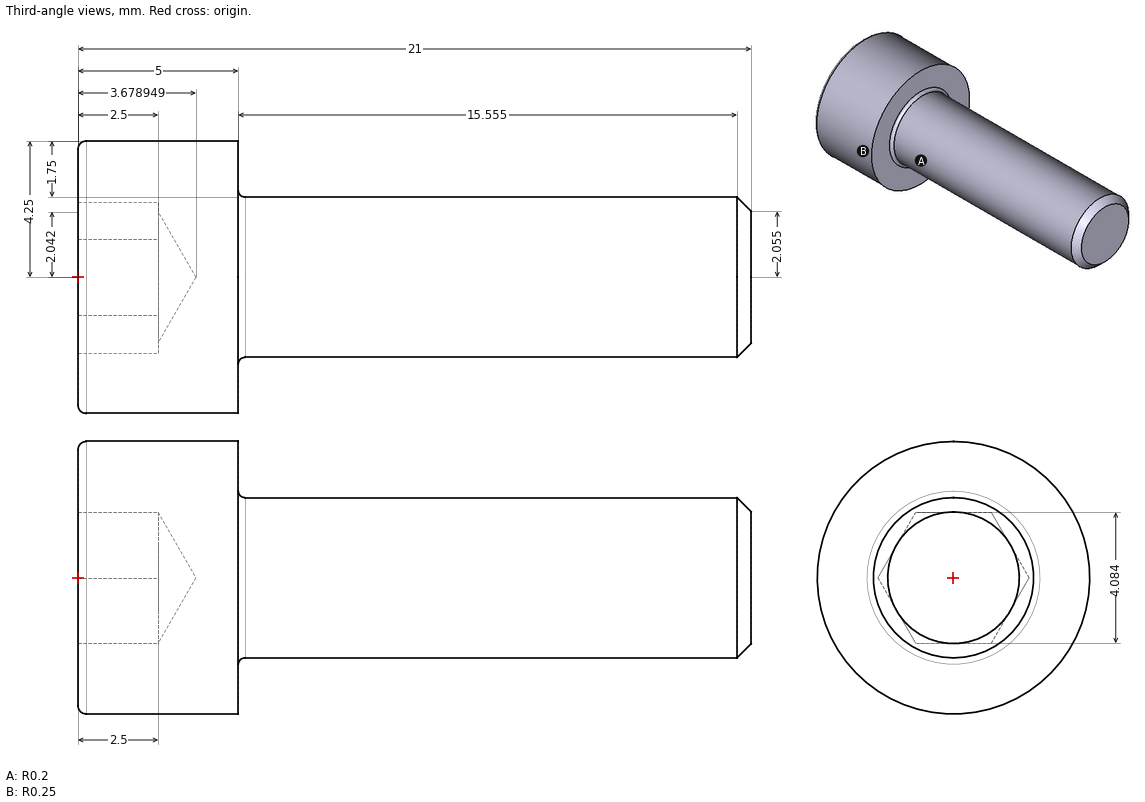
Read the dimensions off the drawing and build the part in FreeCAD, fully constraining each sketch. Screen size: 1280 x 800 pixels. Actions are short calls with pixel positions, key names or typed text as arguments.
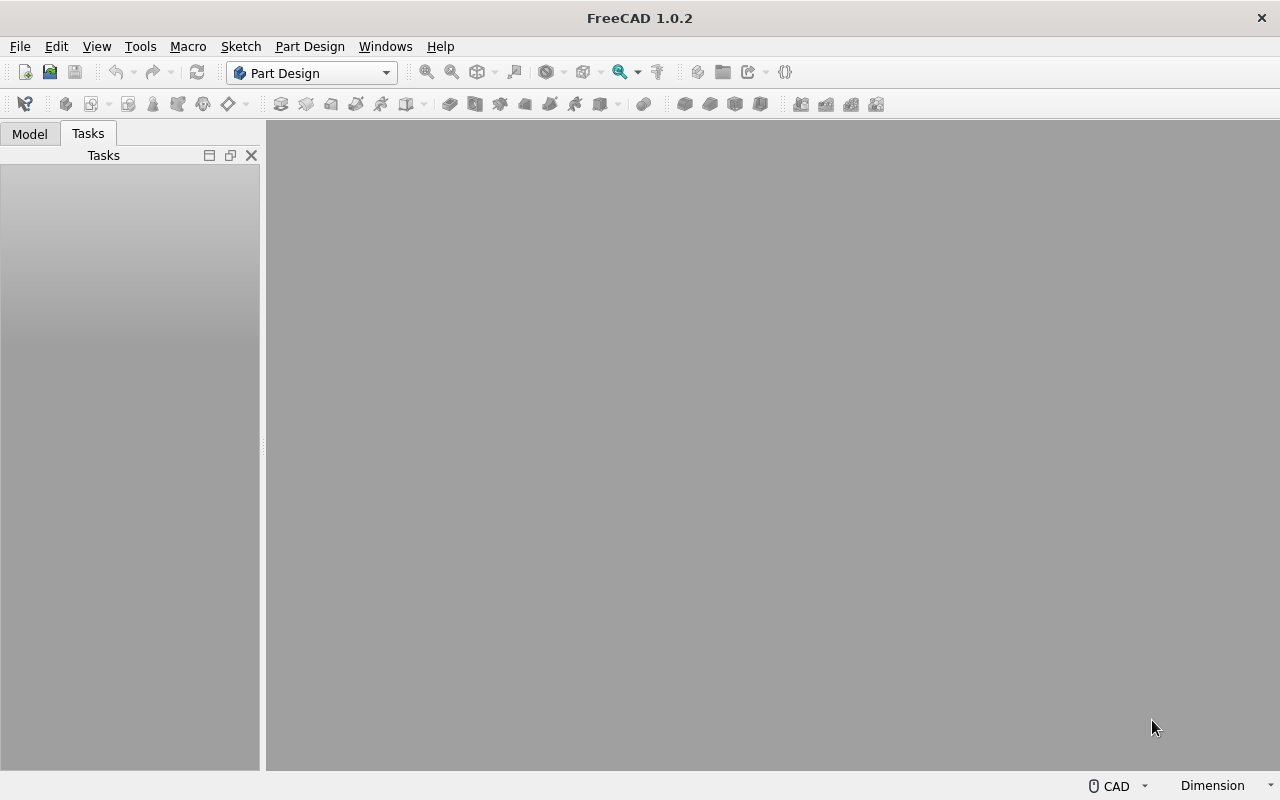
click(25, 72)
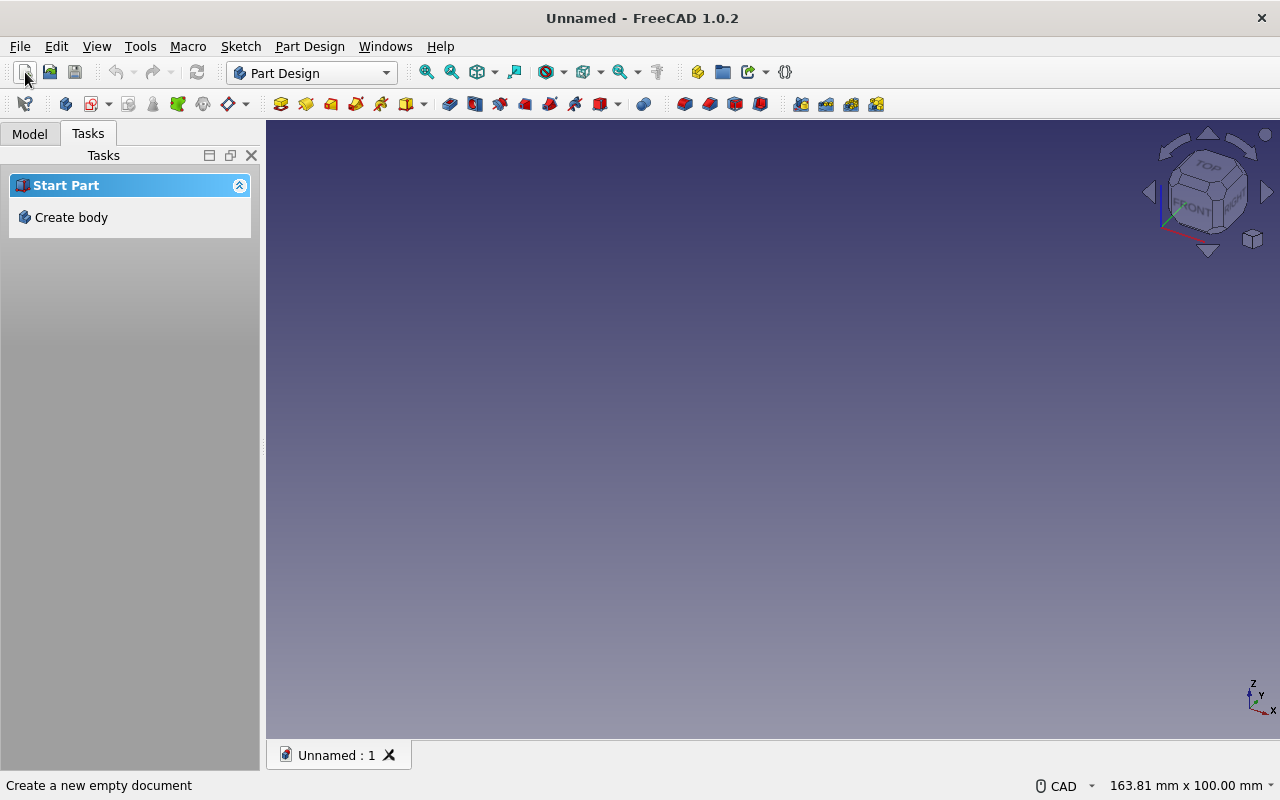
click(90, 104)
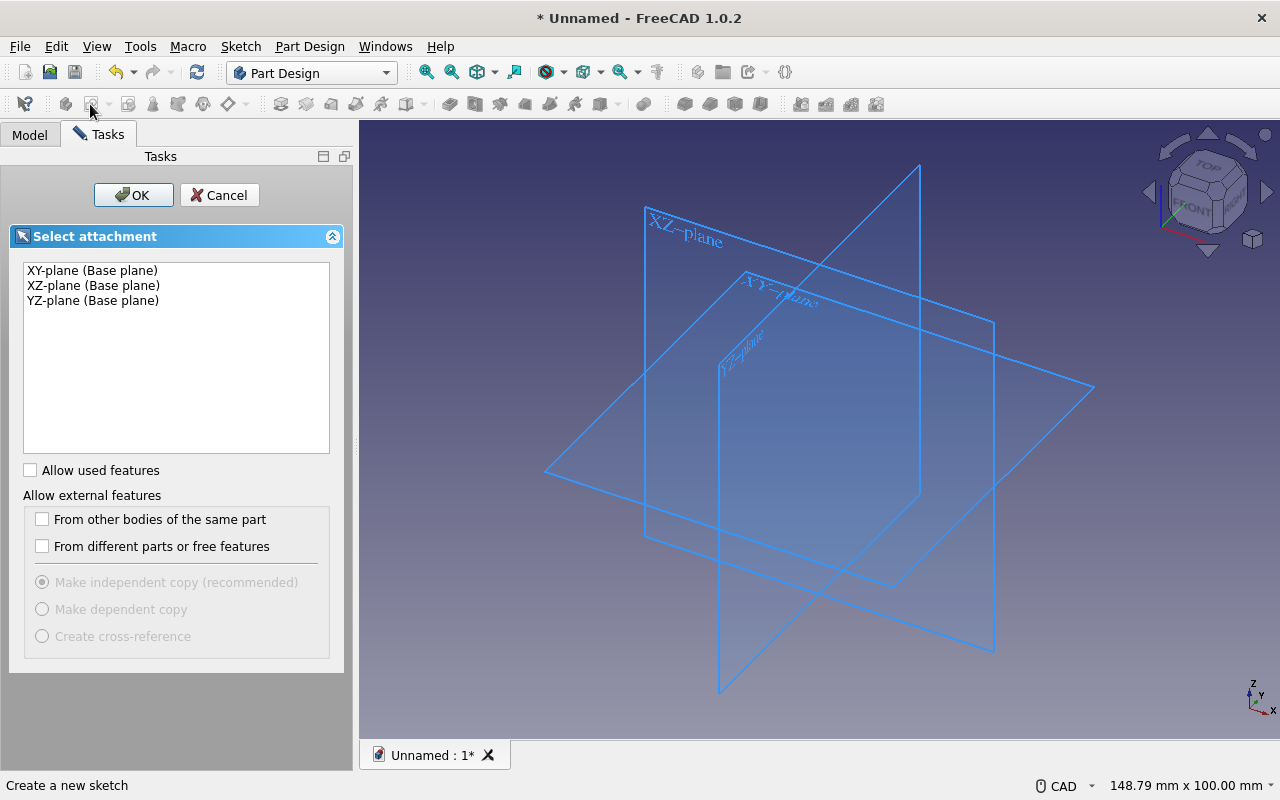
click(84, 270)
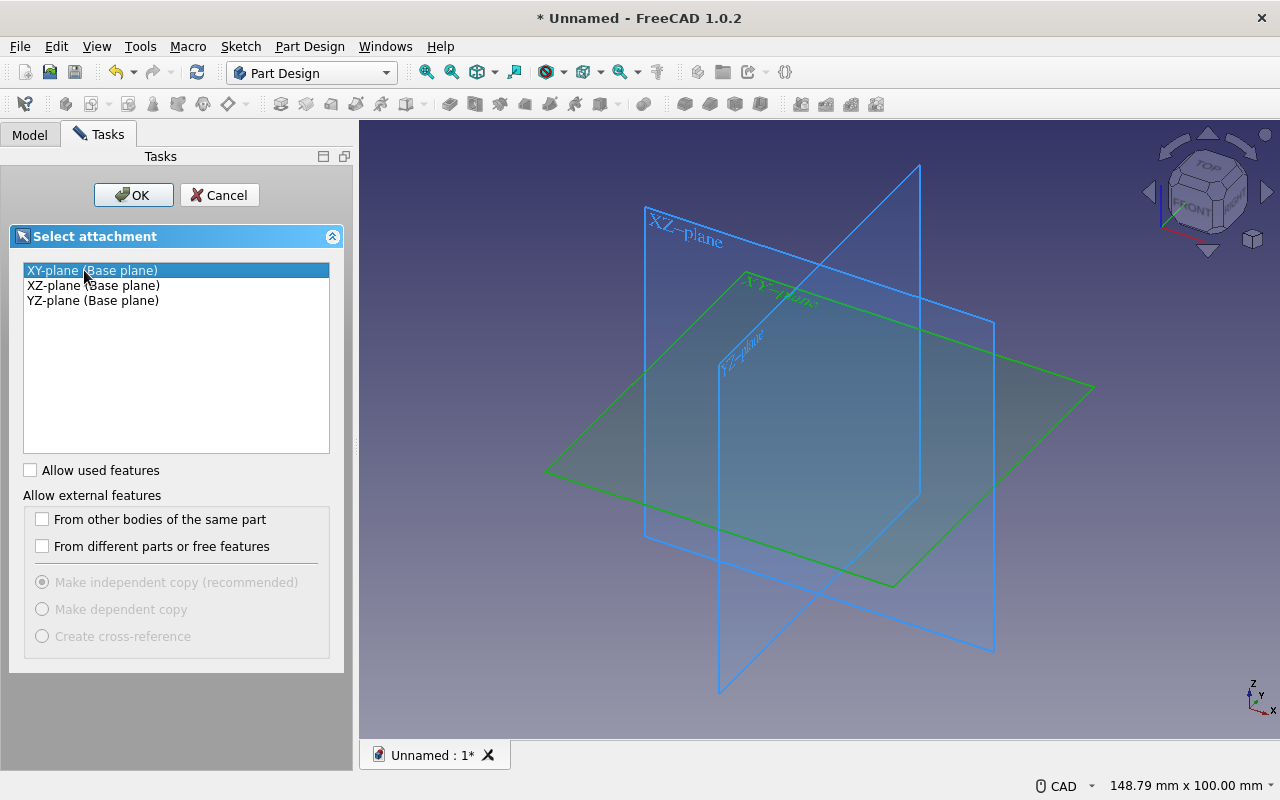
click(134, 195)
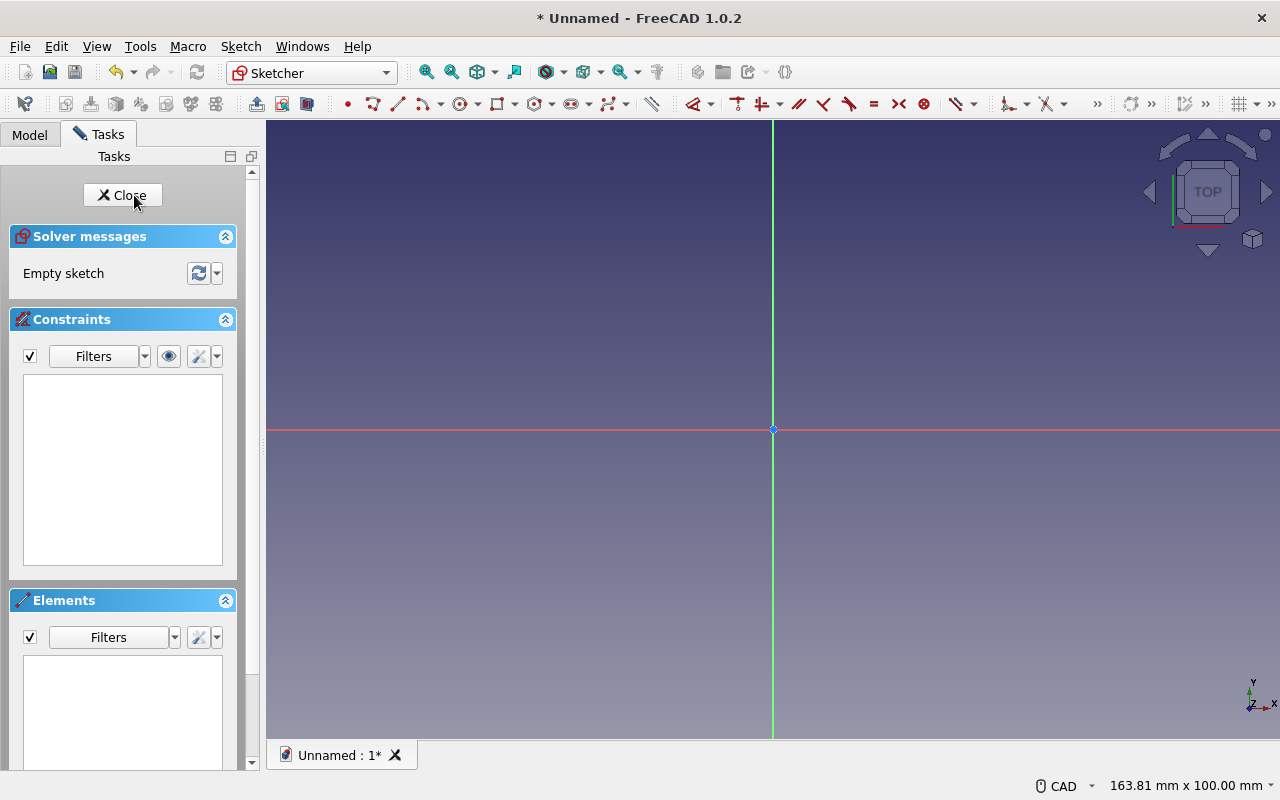
scroll(882, 412, up, 7)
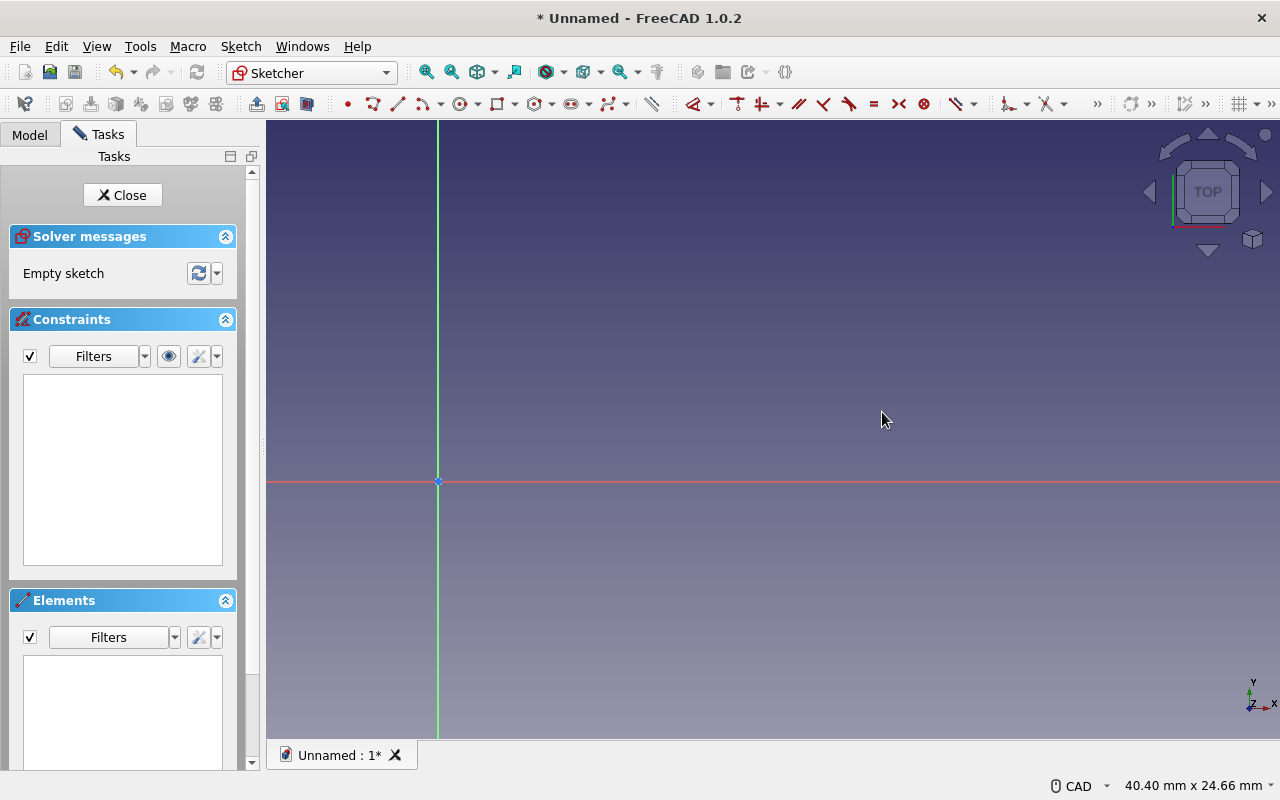
click(373, 104)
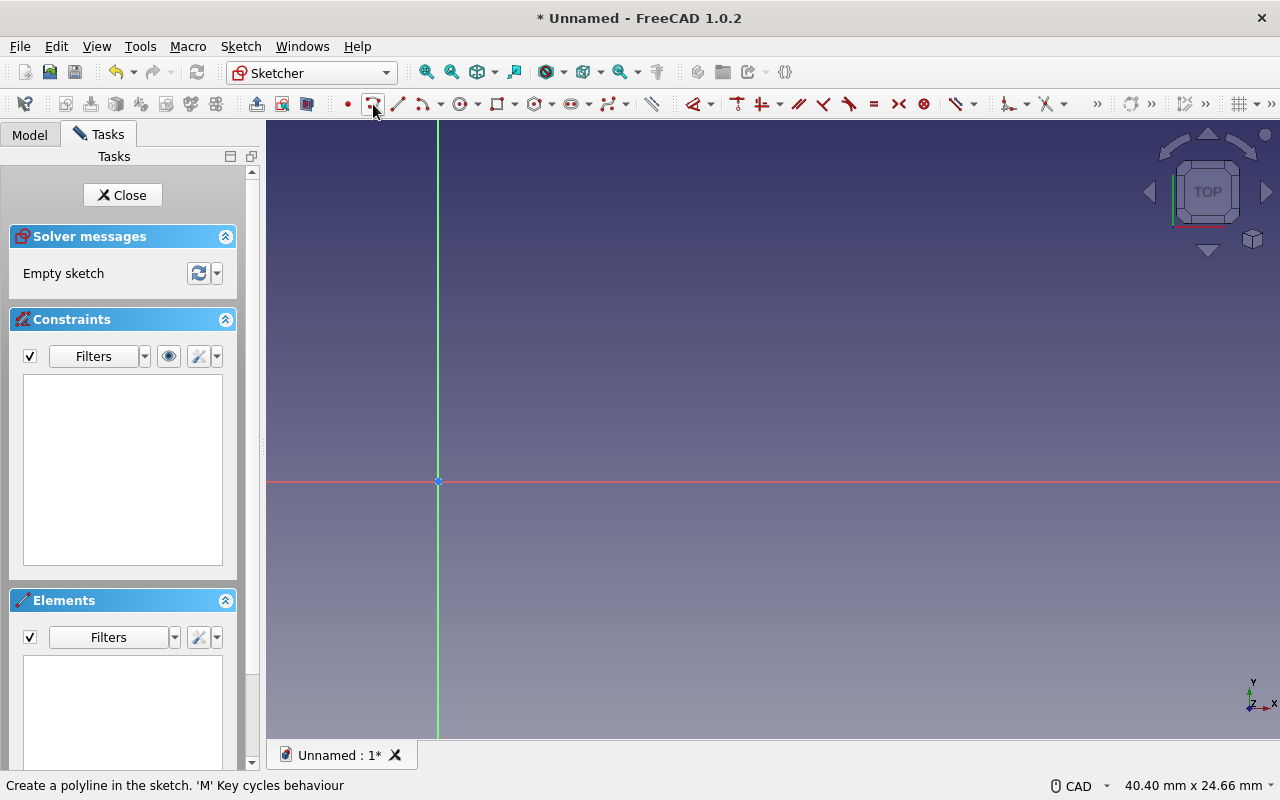
click(438, 482)
click(965, 473)
click(965, 430)
click(954, 419)
click(564, 419)
click(564, 375)
click(447, 375)
click(438, 482)
key(Escape)
key(Escape)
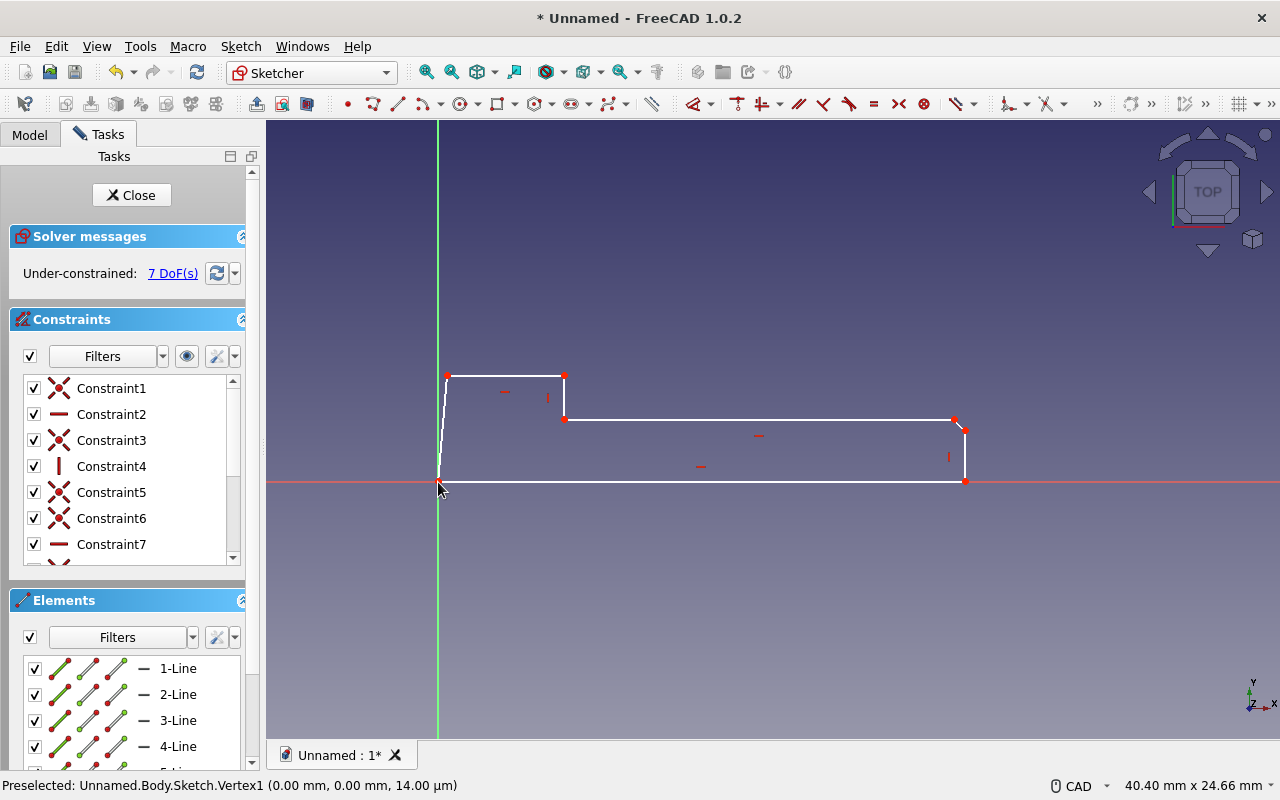
click(441, 450)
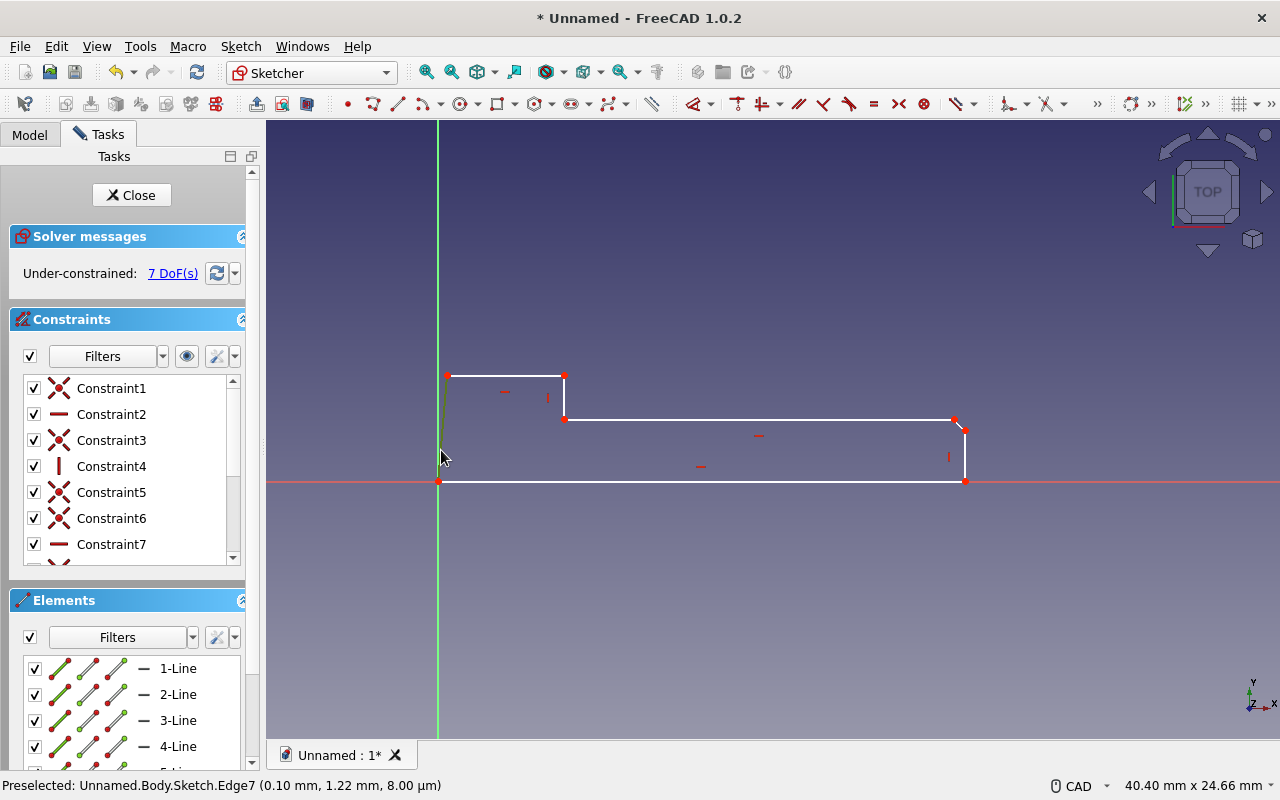
click(780, 104)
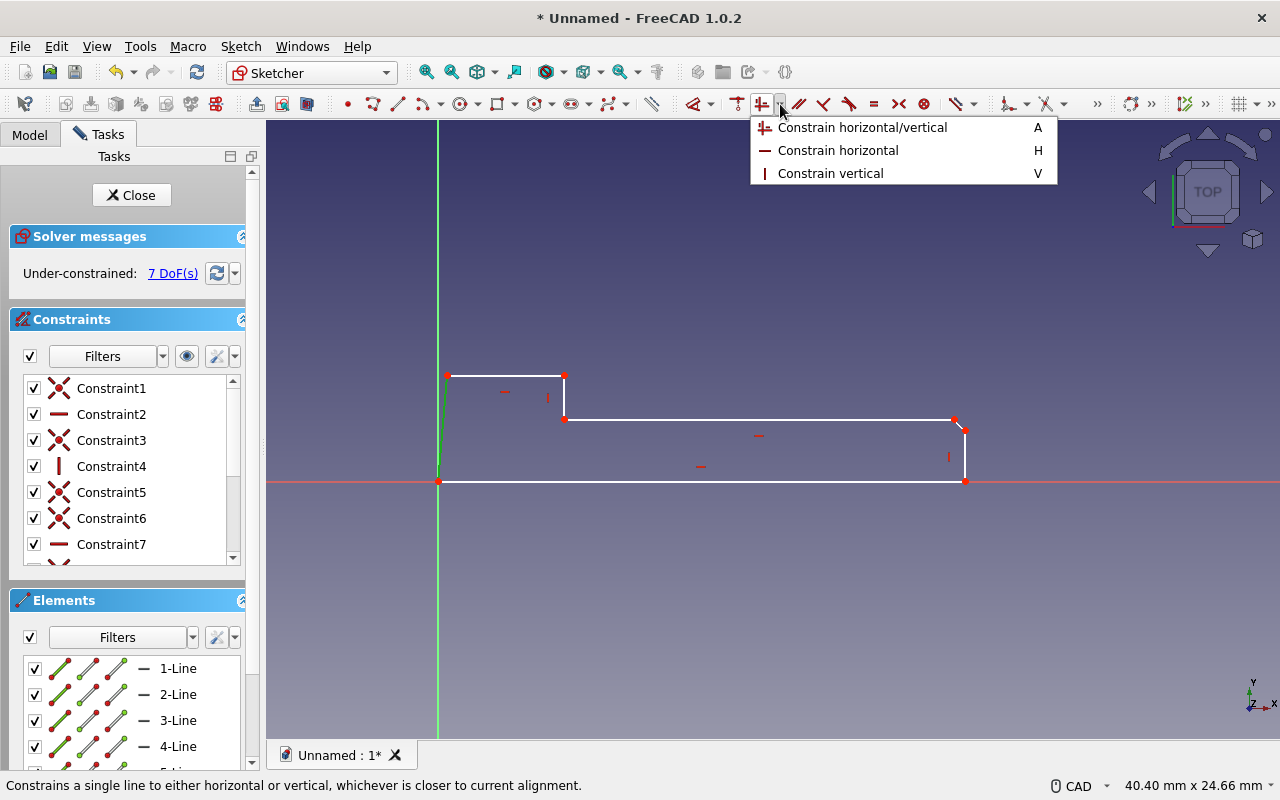
click(904, 174)